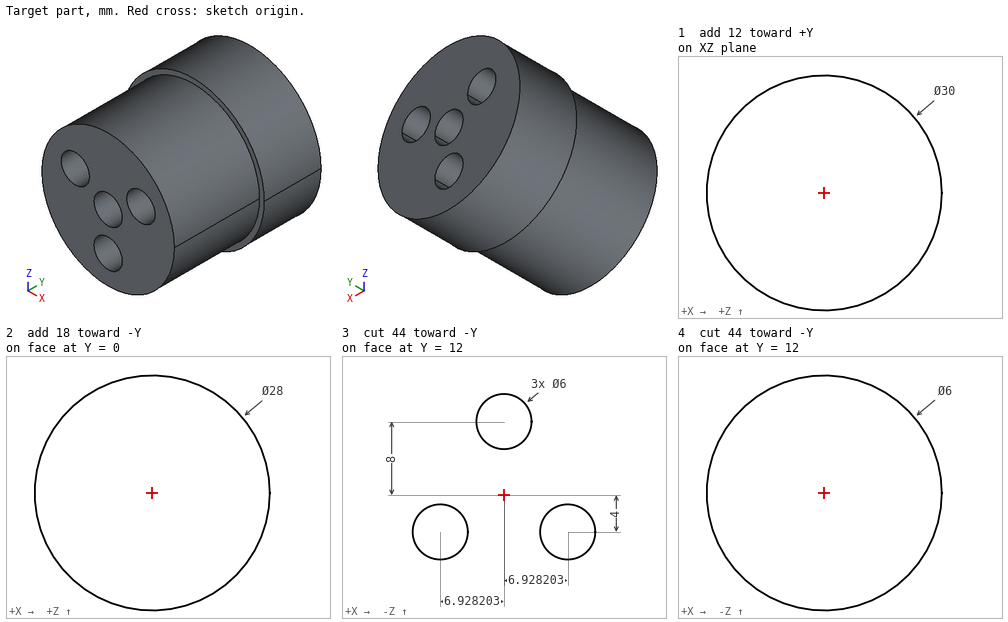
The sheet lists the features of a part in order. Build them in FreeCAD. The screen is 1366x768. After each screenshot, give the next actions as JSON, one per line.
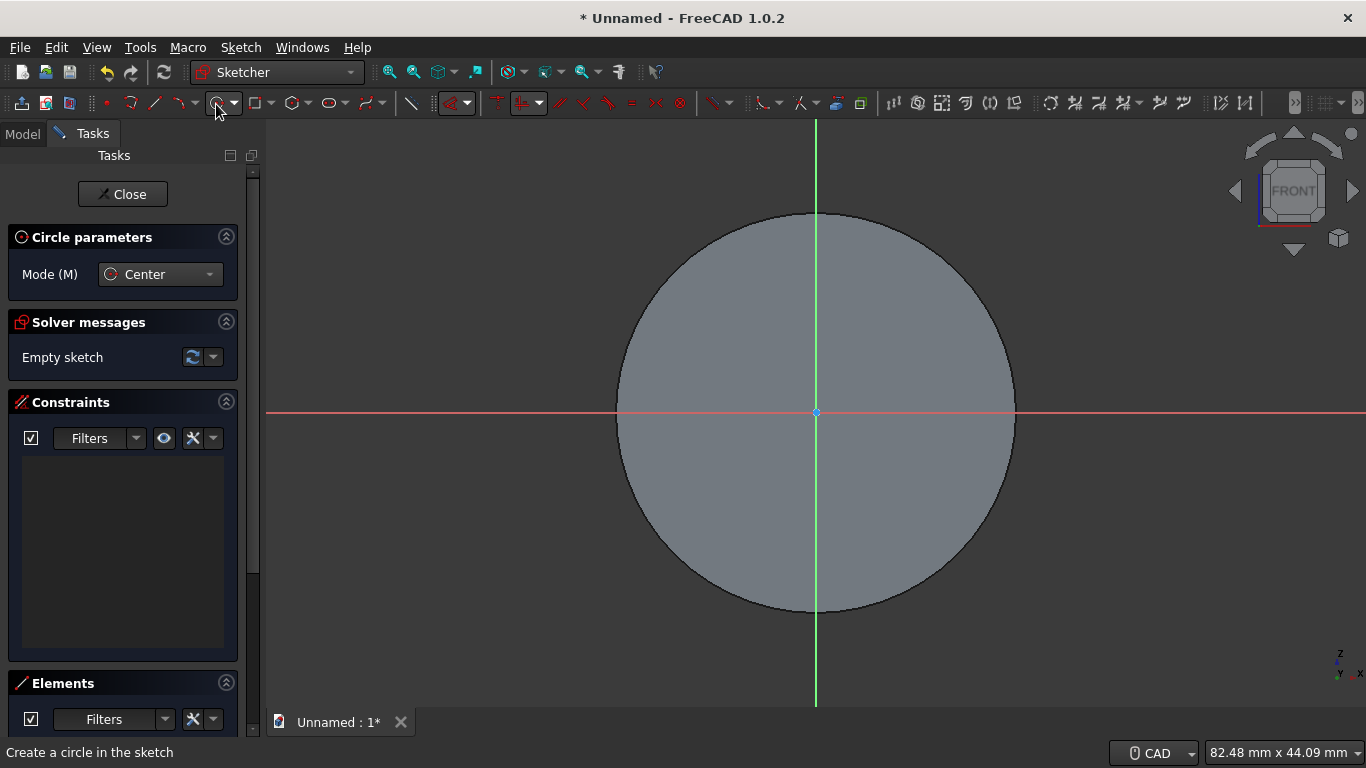
{"action": "left_click", "coordinate": [816, 413]}
{"action": "left_click", "coordinate": [948, 281]}
{"action": "key", "text": "Escape"}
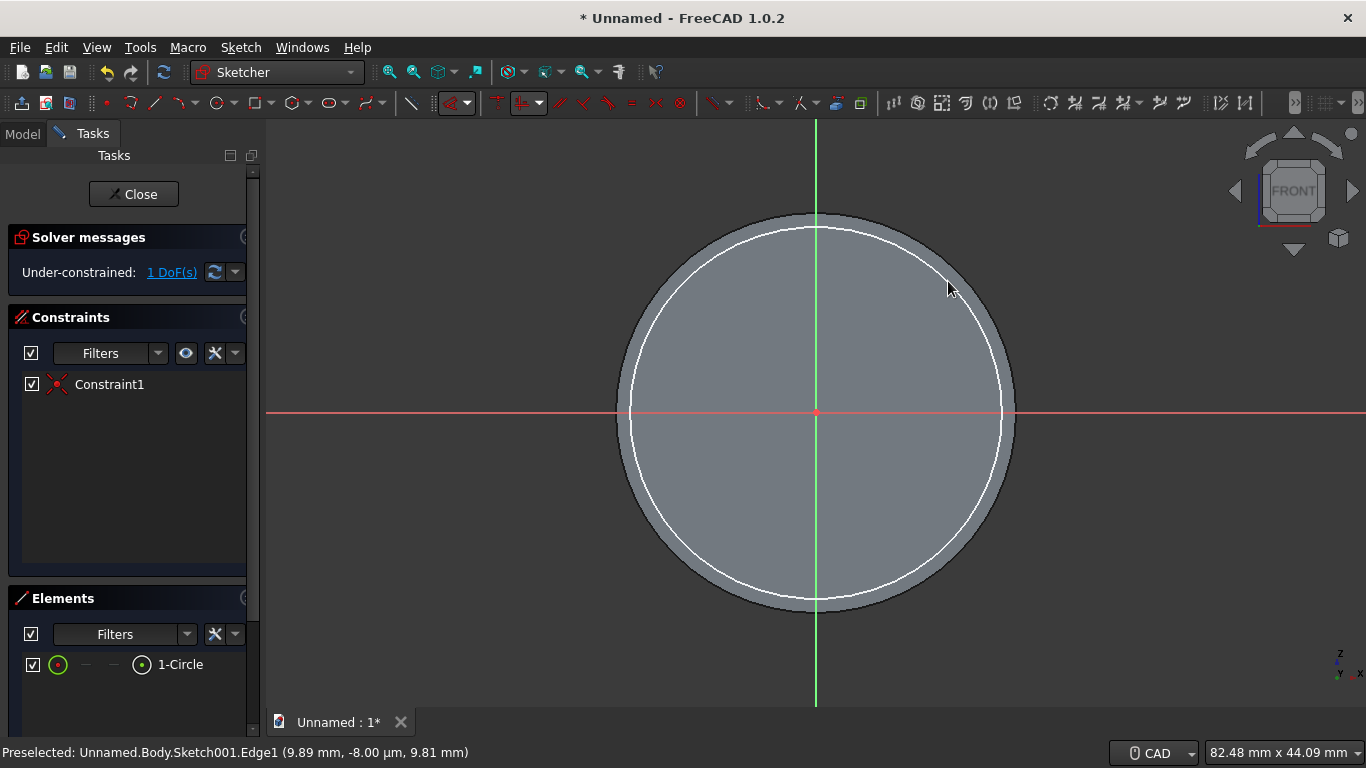
{"action": "left_click", "coordinate": [947, 281]}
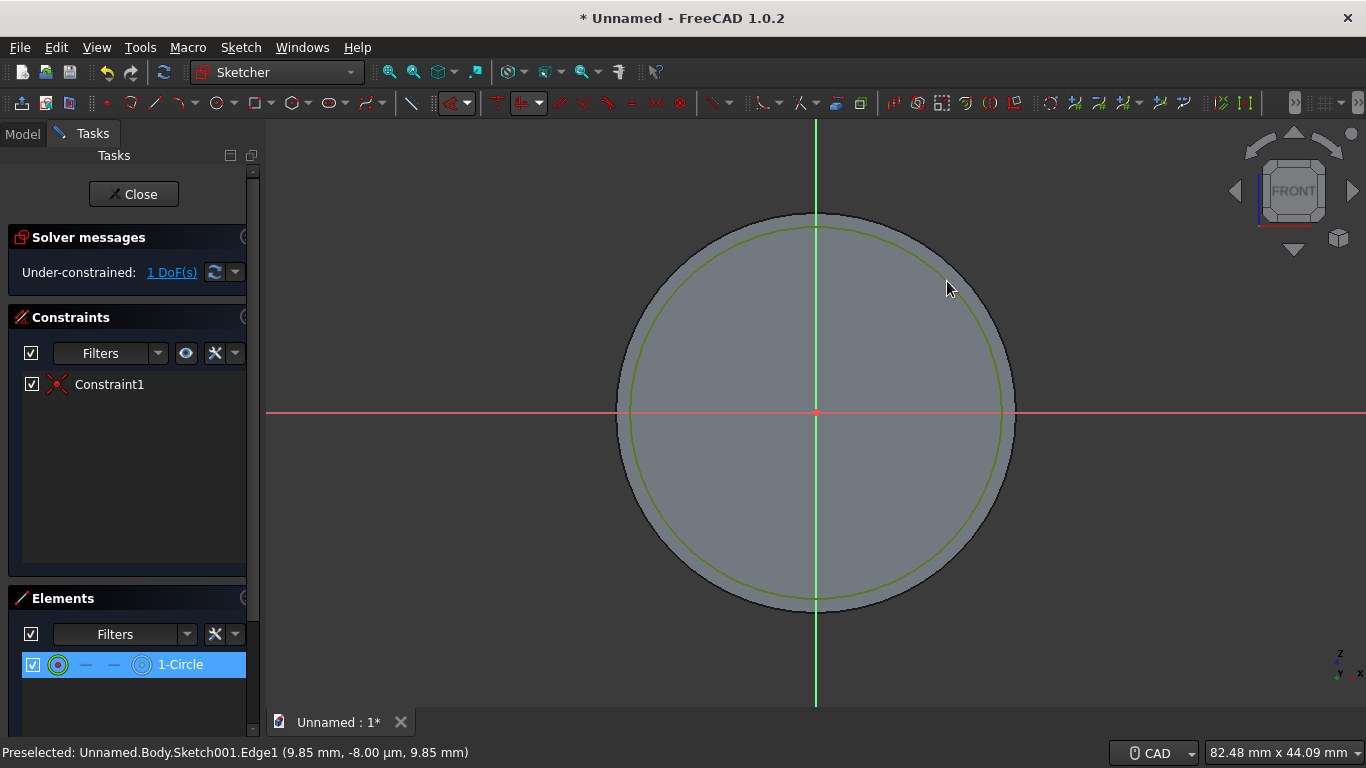
{"action": "left_click", "coordinate": [470, 104]}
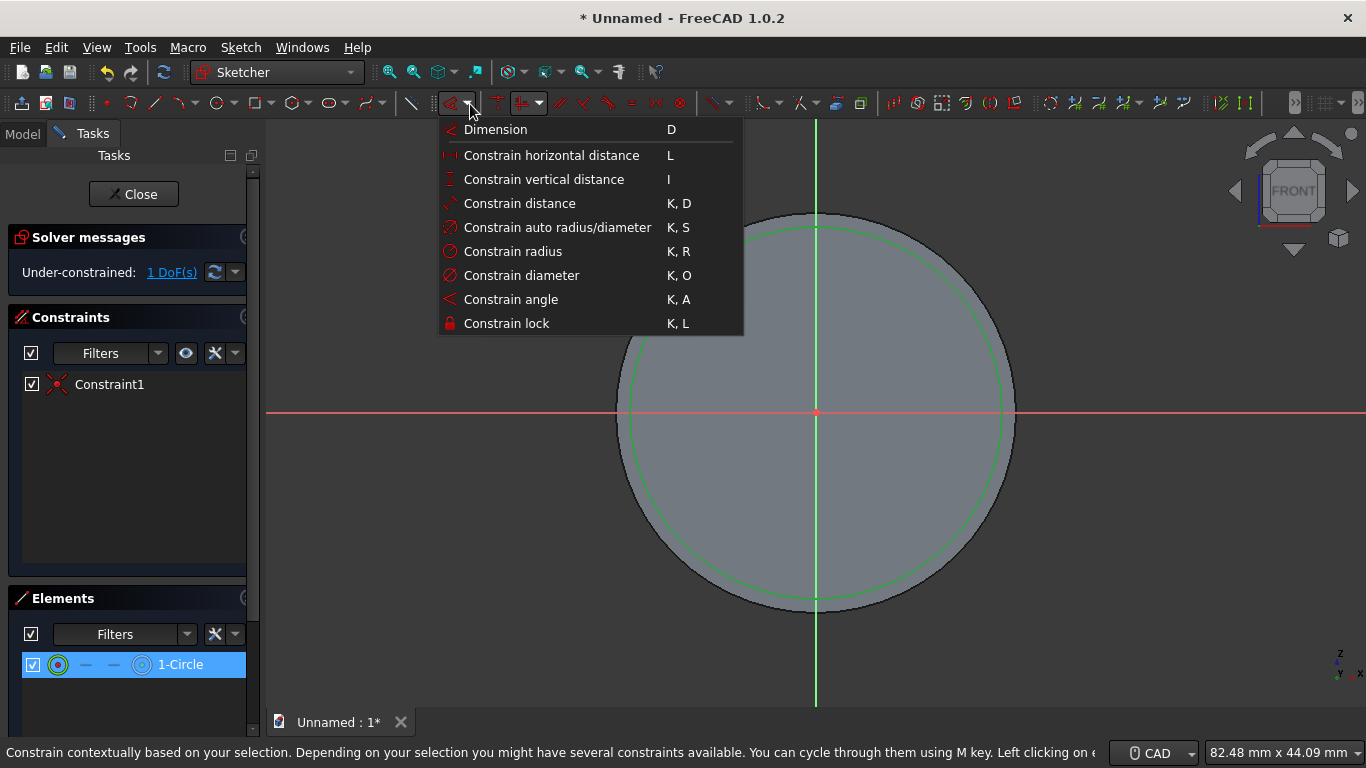
{"action": "left_click", "coordinate": [591, 275]}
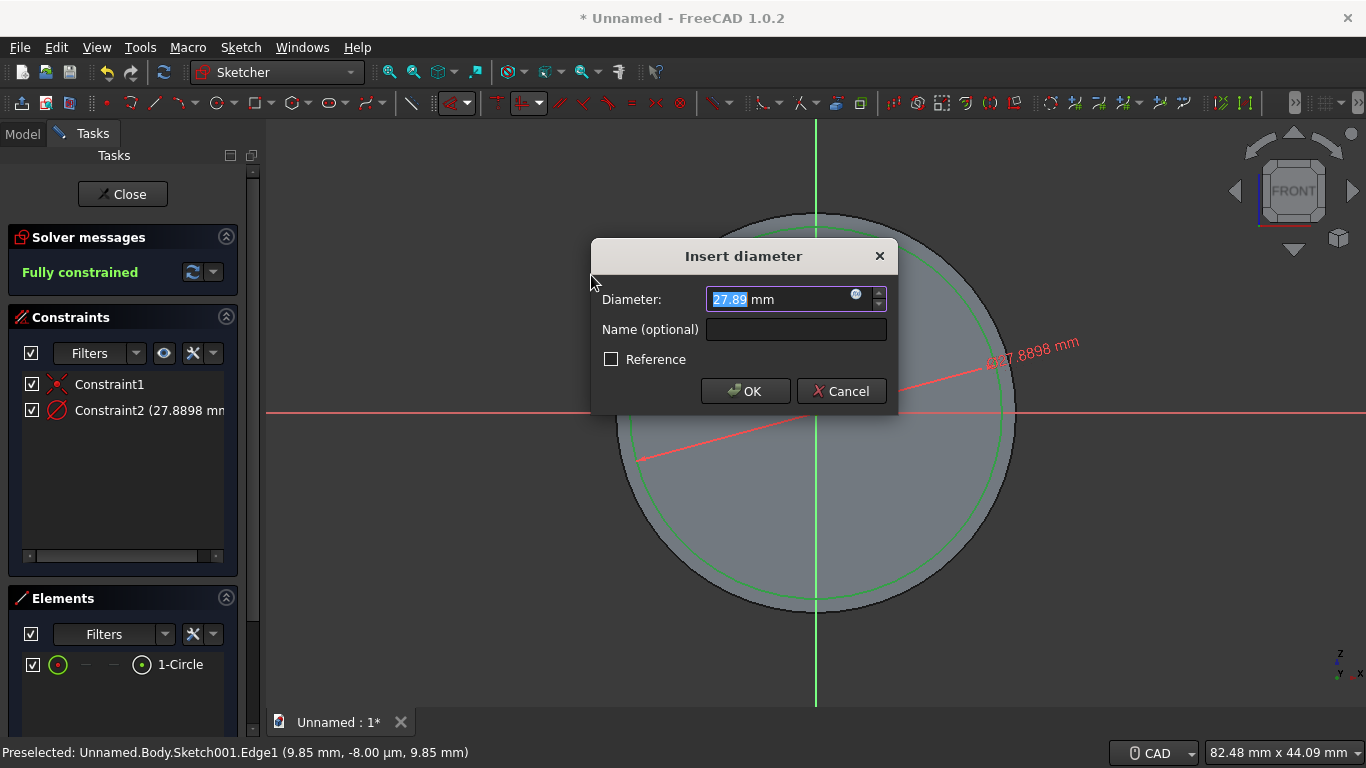
{"action": "type", "text": "28"}
{"action": "key", "text": "Return"}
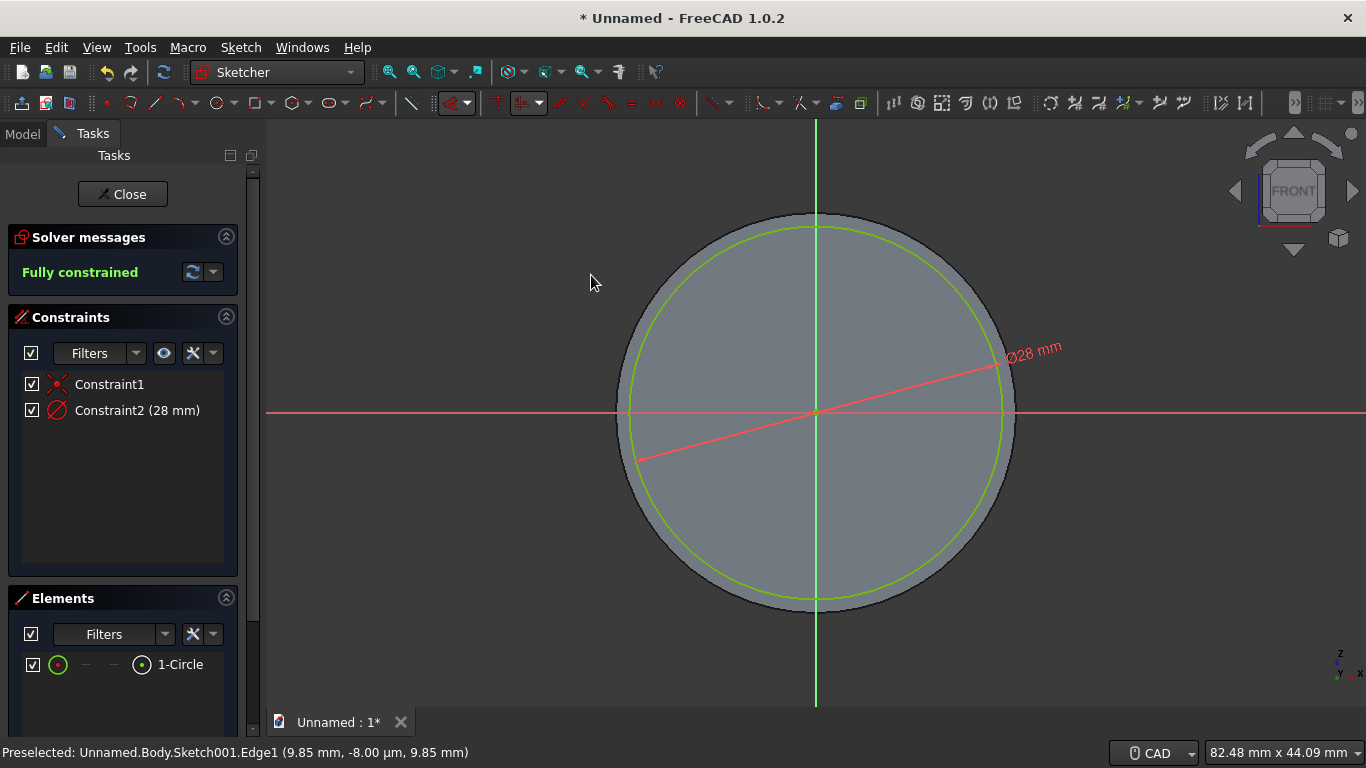
{"action": "left_click", "coordinate": [123, 194]}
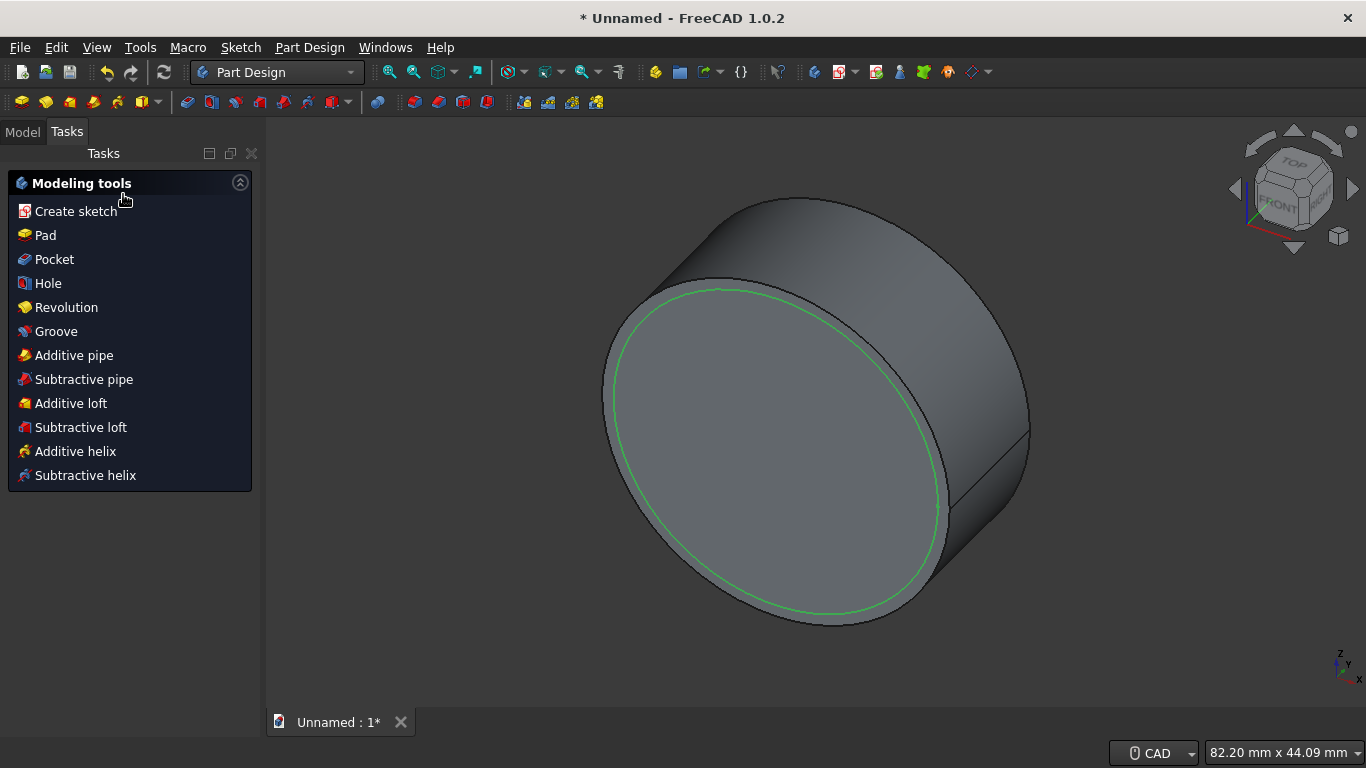
{"action": "left_click", "coordinate": [22, 102]}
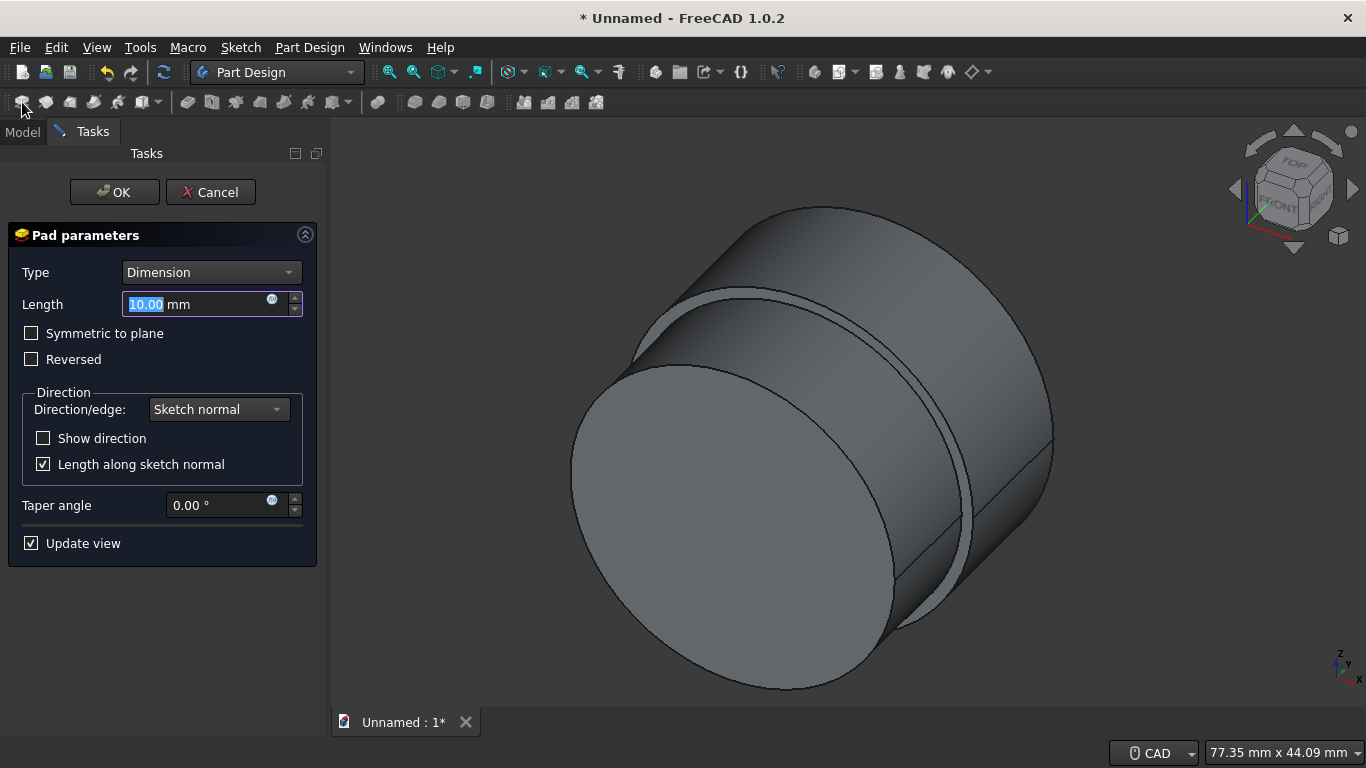
{"action": "type", "text": "18"}
{"action": "key", "text": "Tab"}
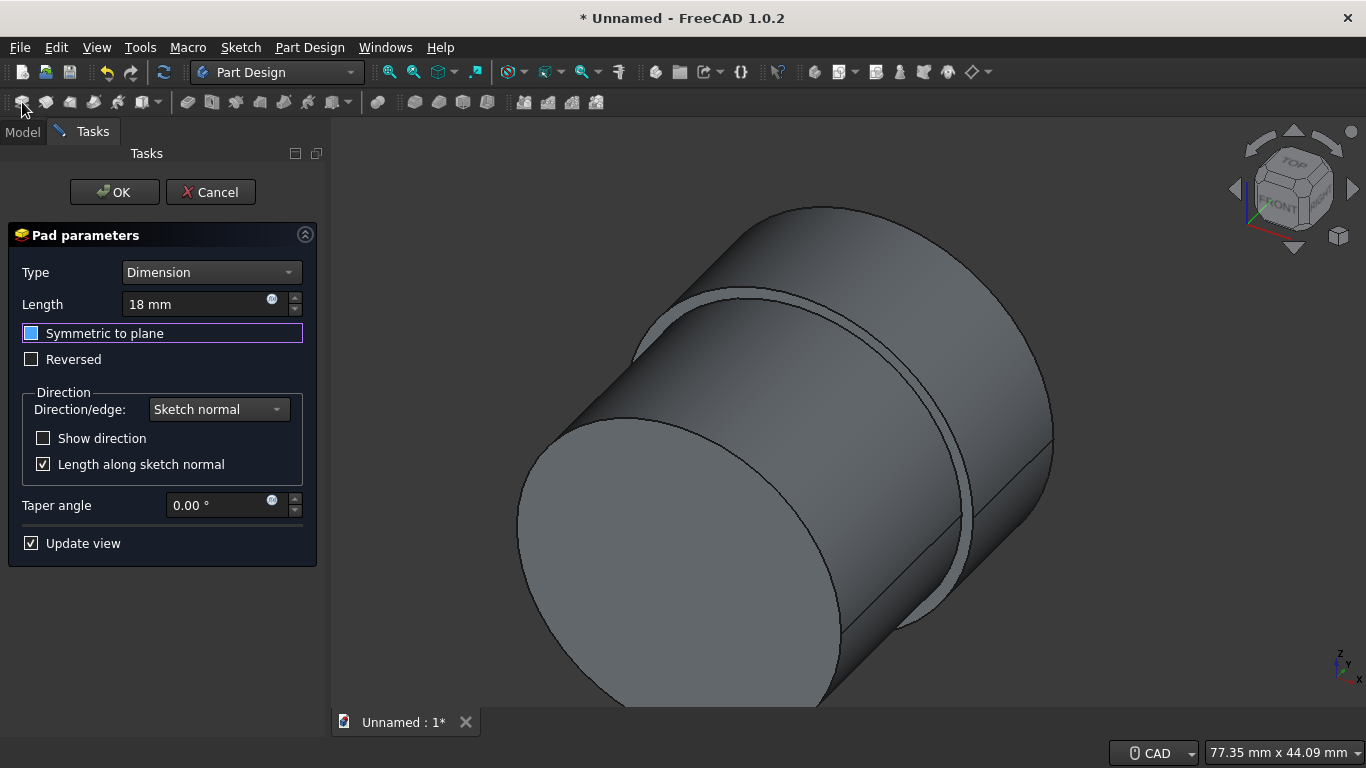
{"action": "left_click", "coordinate": [115, 192]}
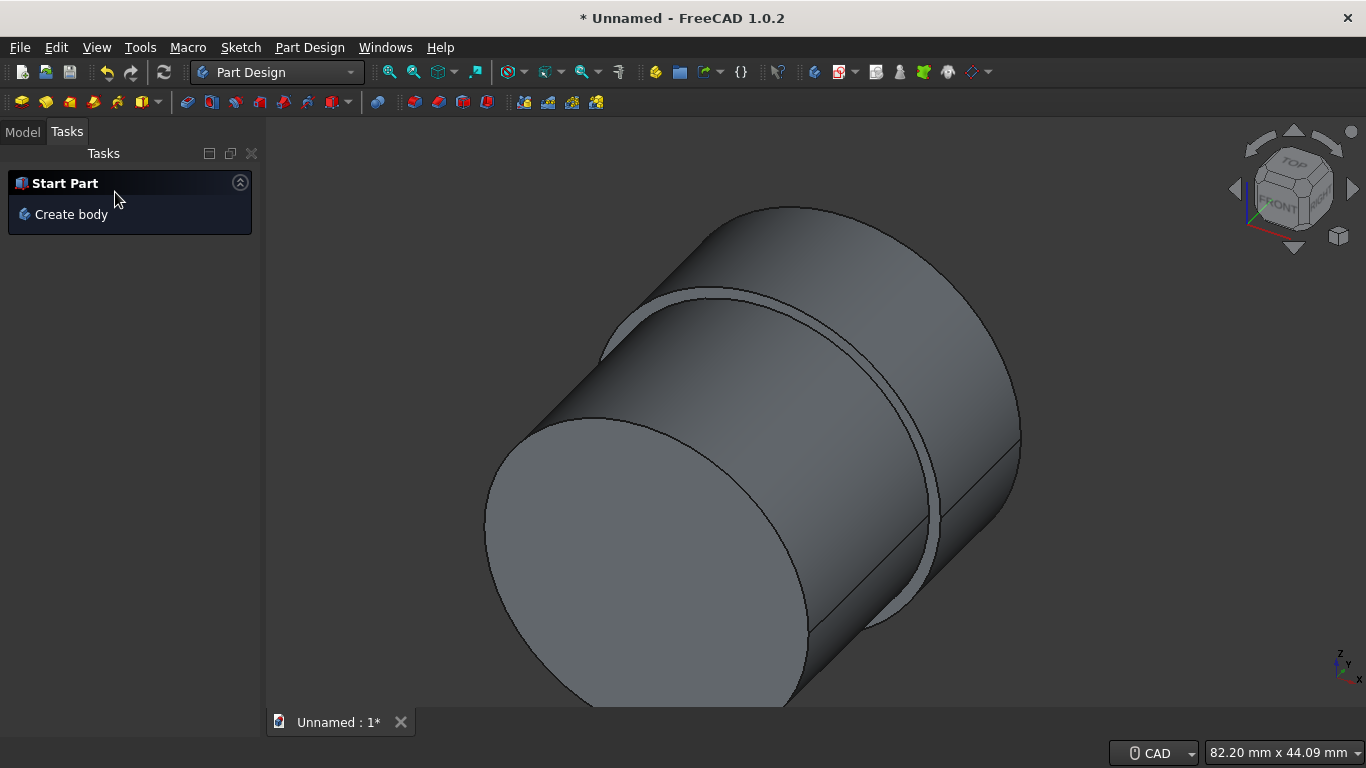
{"action": "left_click", "coordinate": [390, 72]}